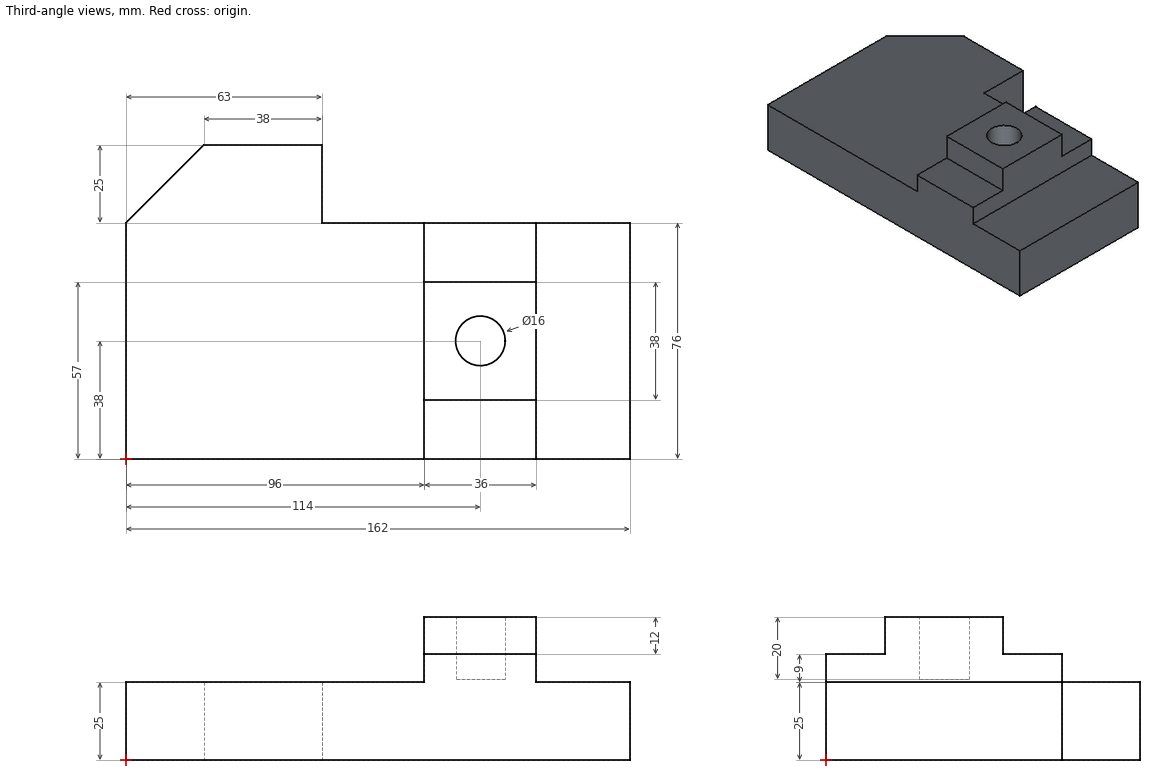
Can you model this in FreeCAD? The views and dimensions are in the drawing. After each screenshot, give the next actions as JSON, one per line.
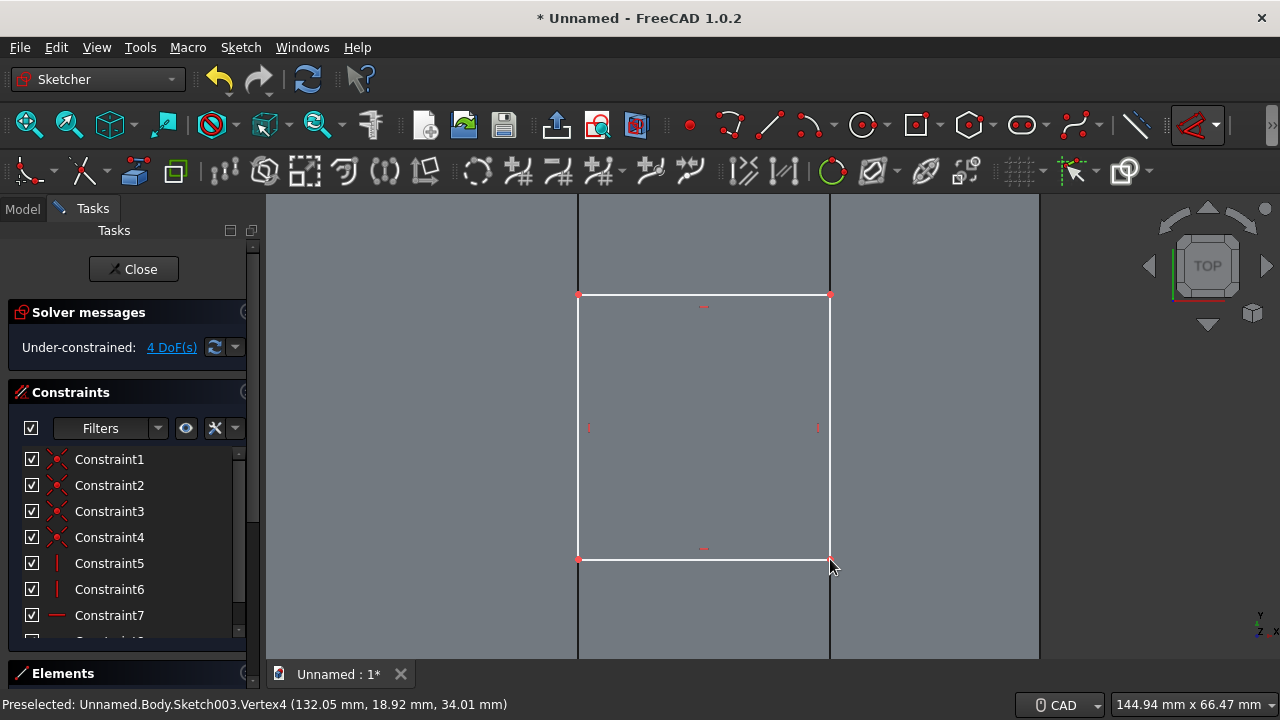
{"action": "left_click", "coordinate": [578, 374]}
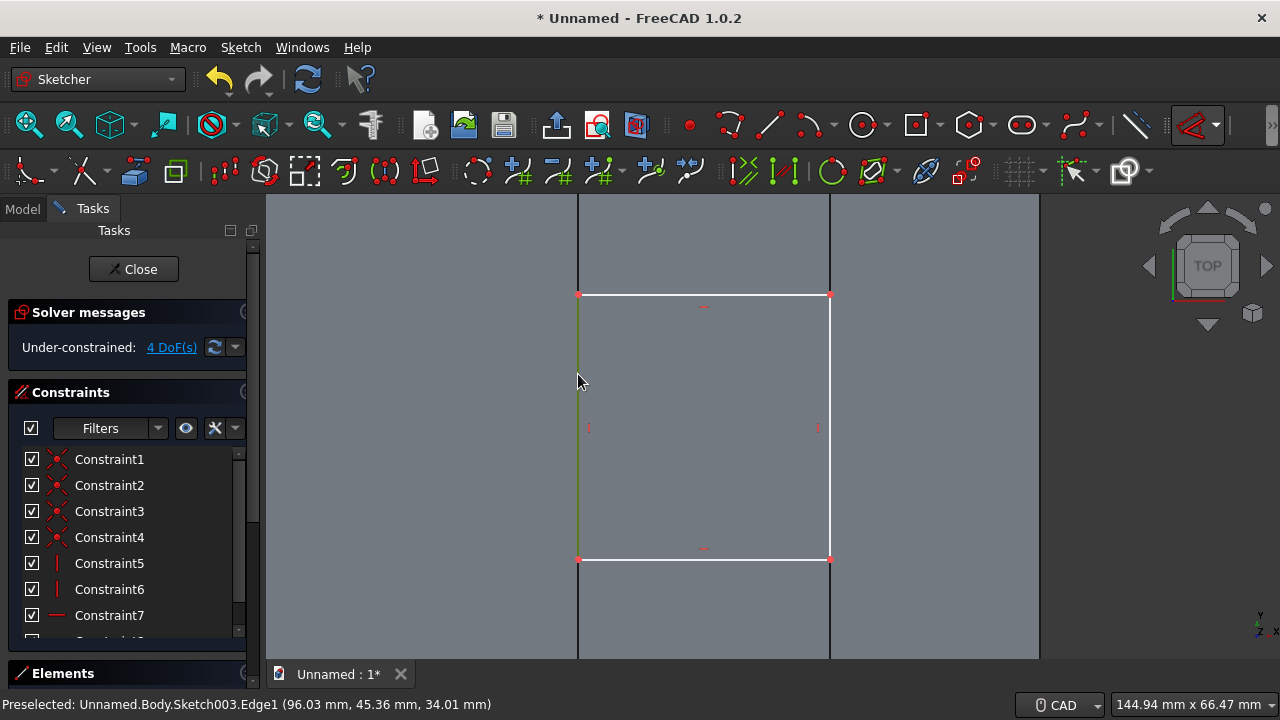
{"action": "key", "text": "i"}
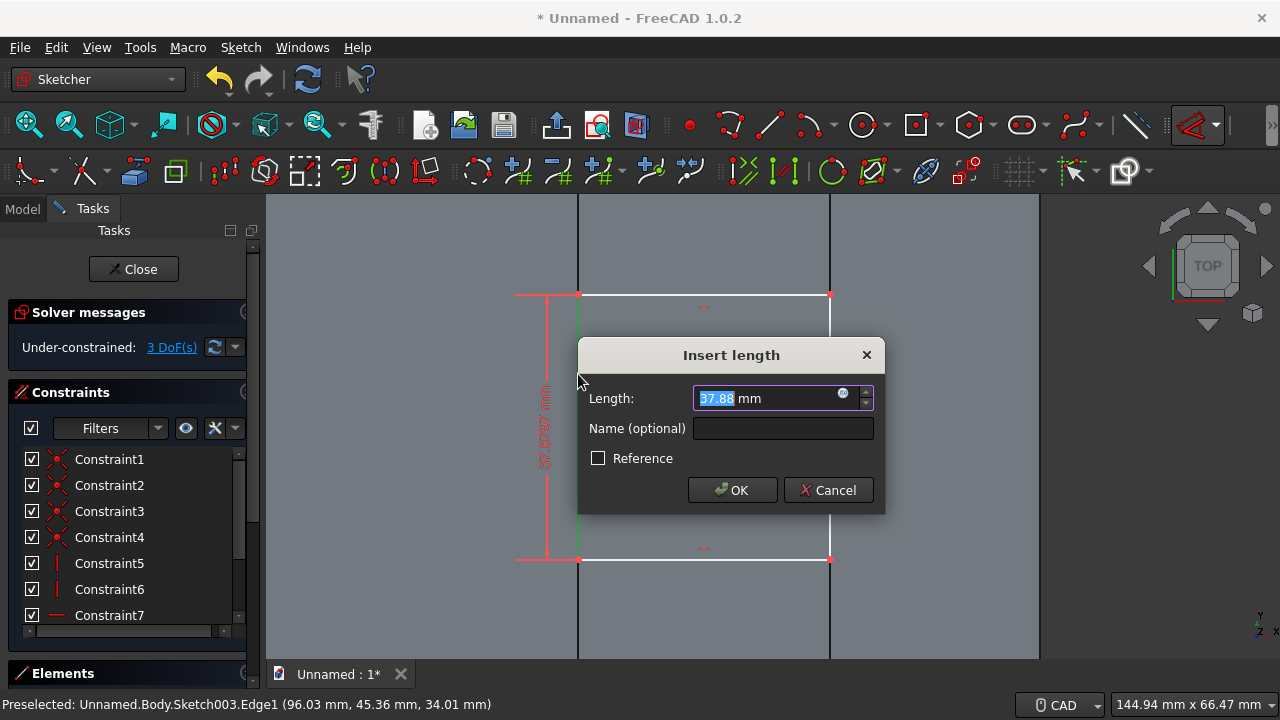
{"action": "type", "text": "38"}
{"action": "key", "text": "Return"}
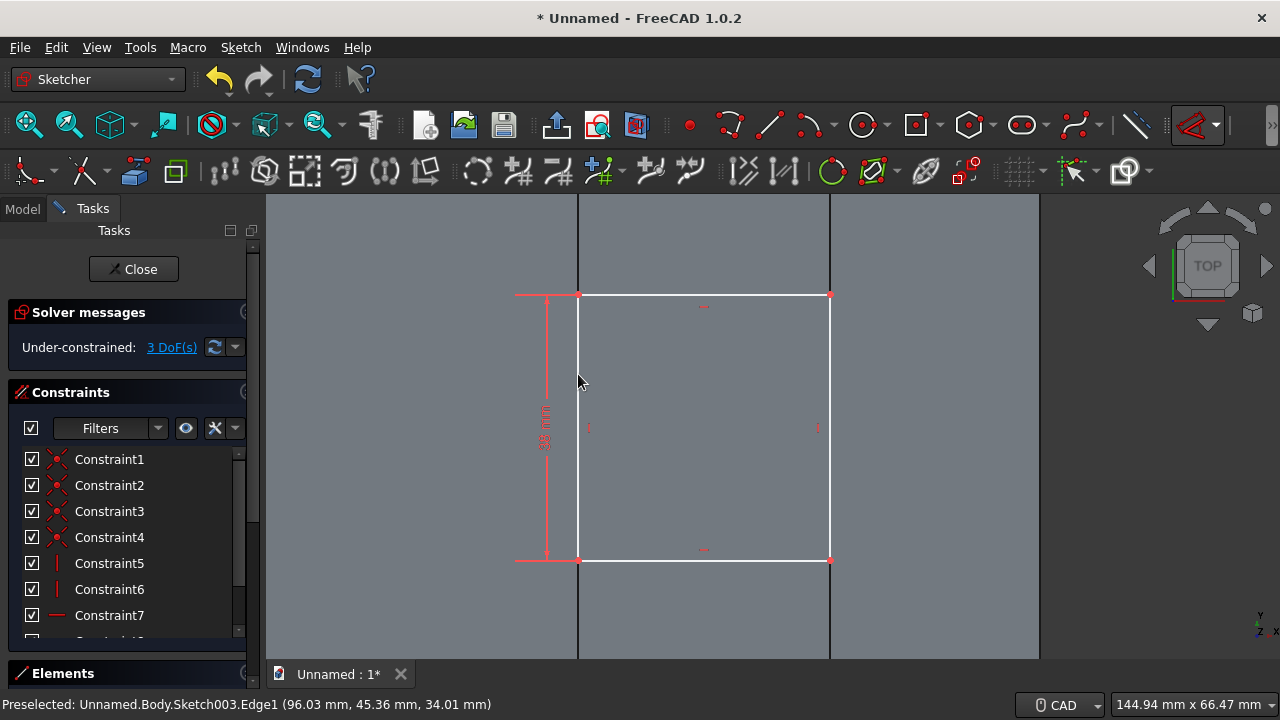
{"action": "left_click", "coordinate": [654, 561]}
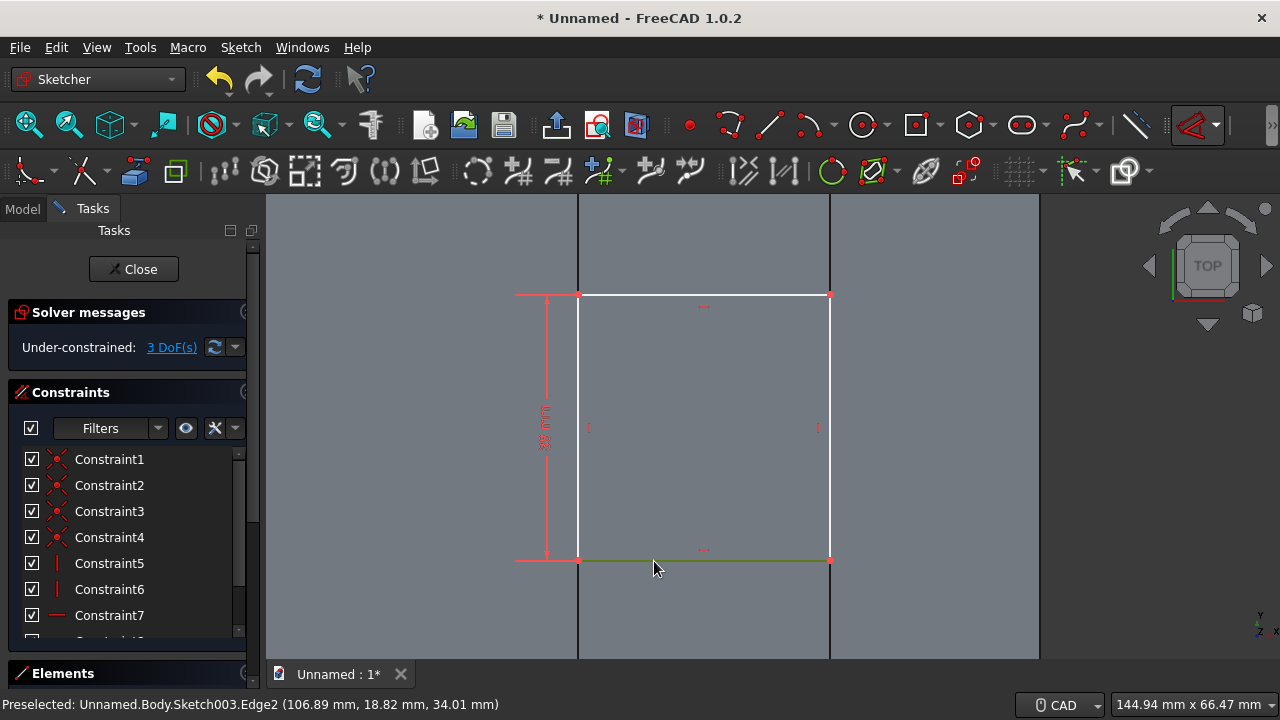
{"action": "key", "text": "l"}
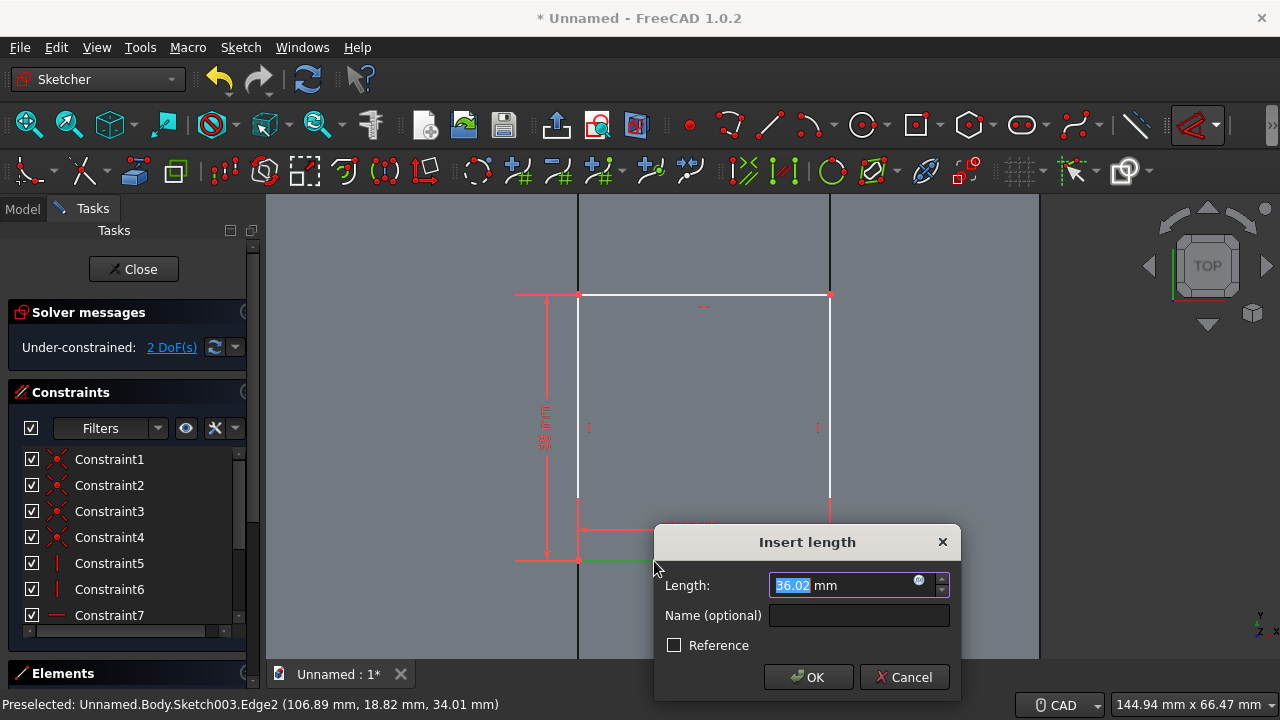
{"action": "type", "text": "36"}
{"action": "key", "text": "Return"}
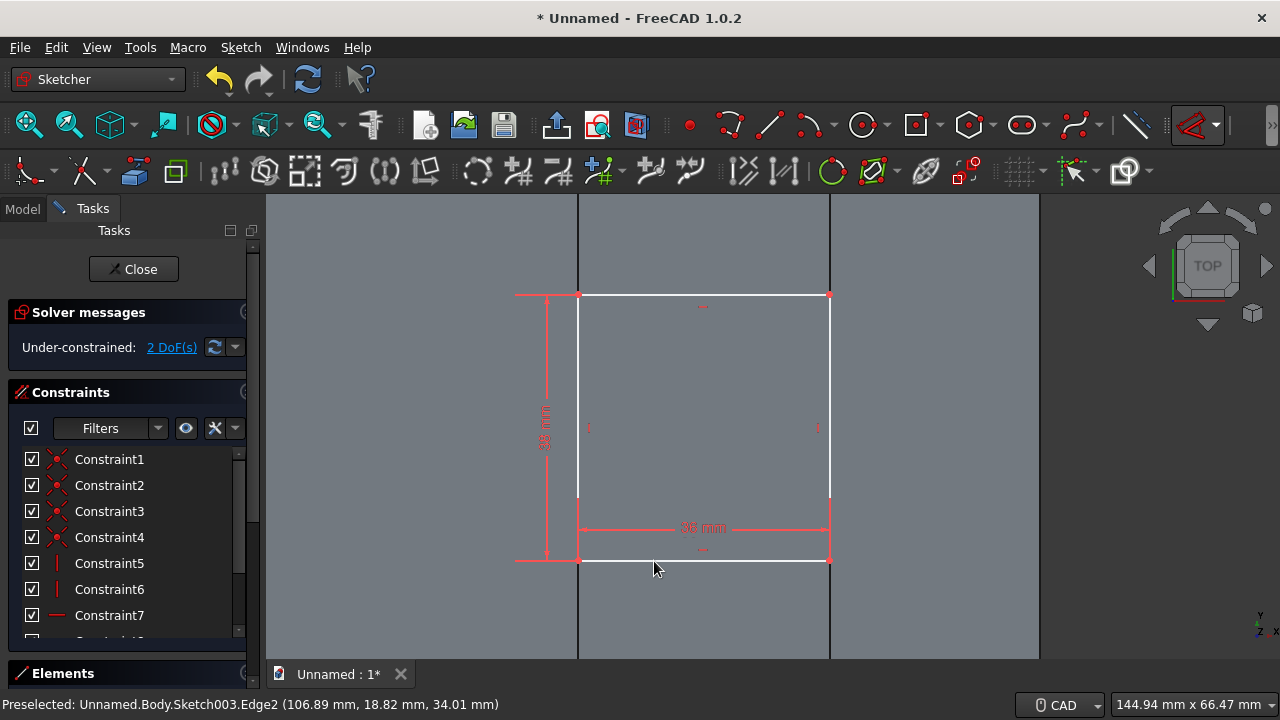
{"action": "left_click", "coordinate": [578, 295]}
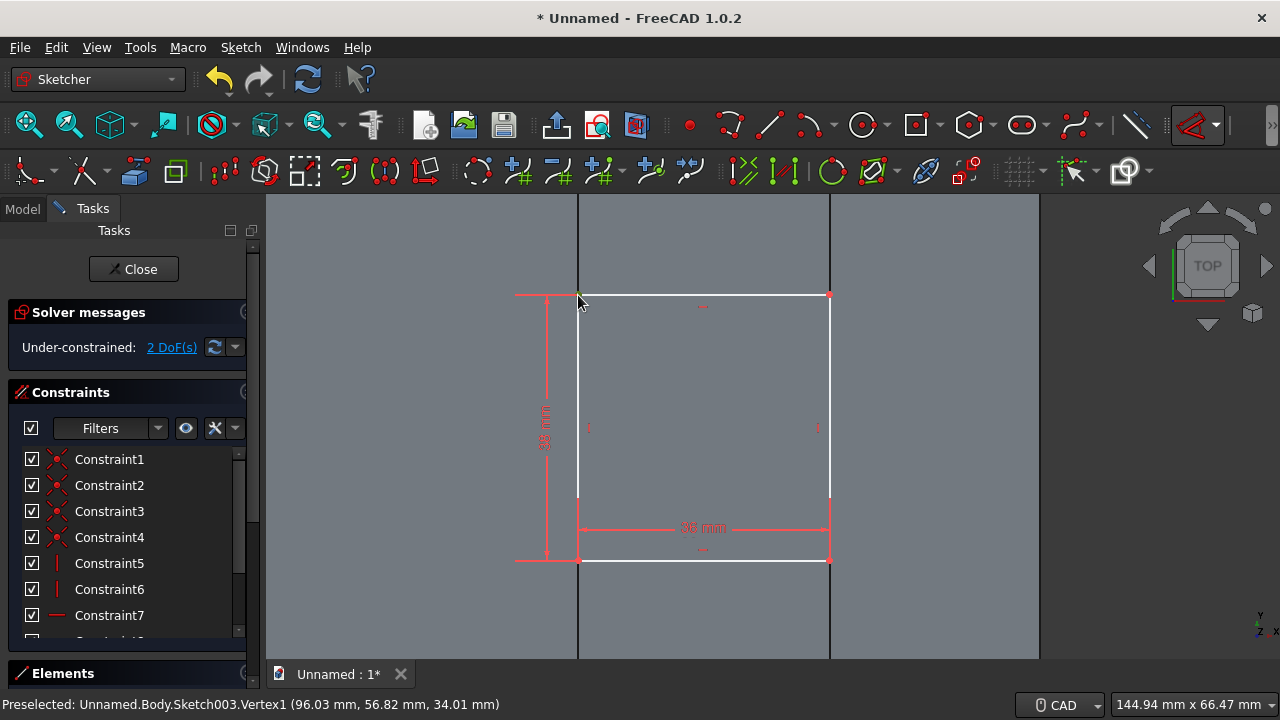
{"action": "key", "text": "l"}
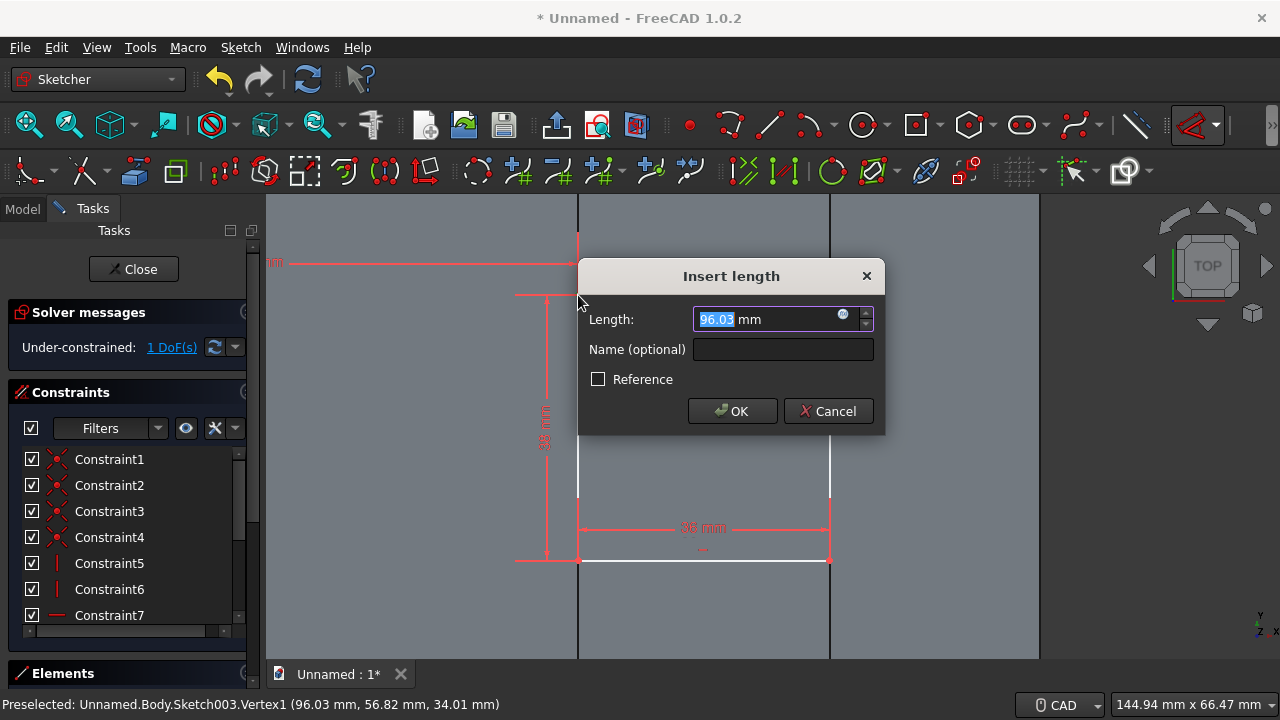
{"action": "type", "text": "96"}
{"action": "key", "text": "Return"}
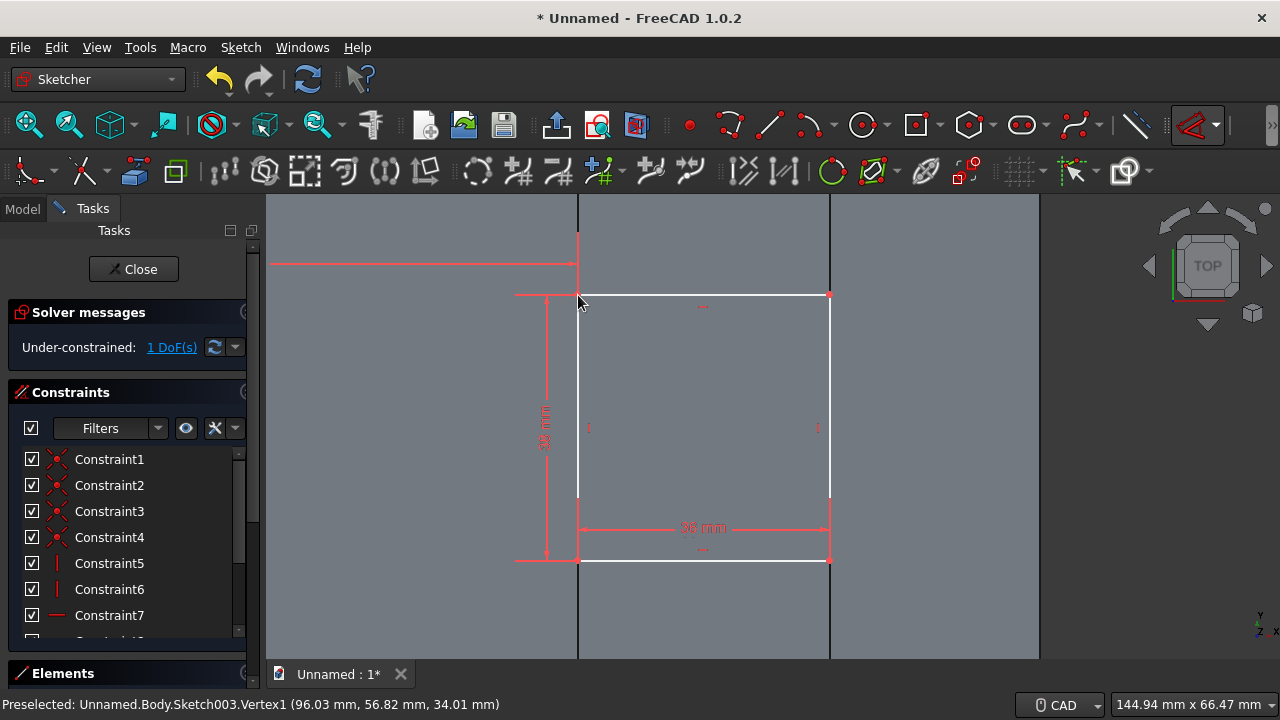
{"action": "left_click", "coordinate": [578, 295]}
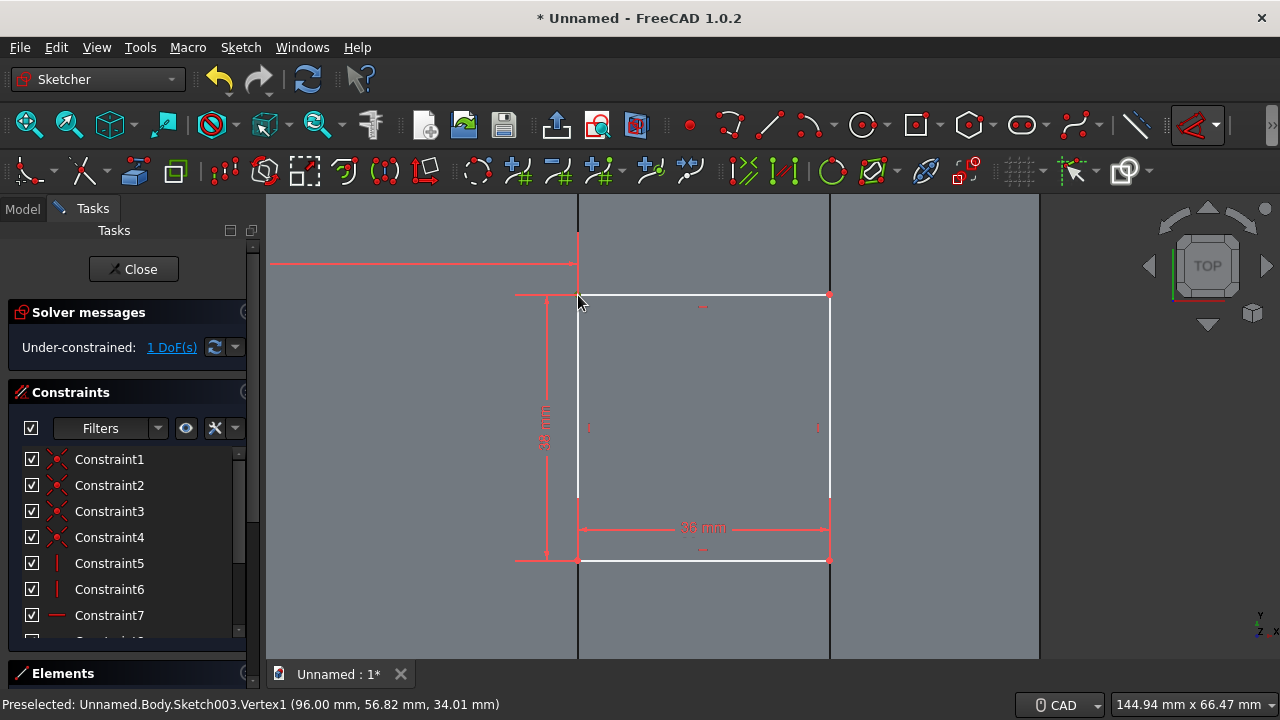
{"action": "left_click", "coordinate": [1218, 126]}